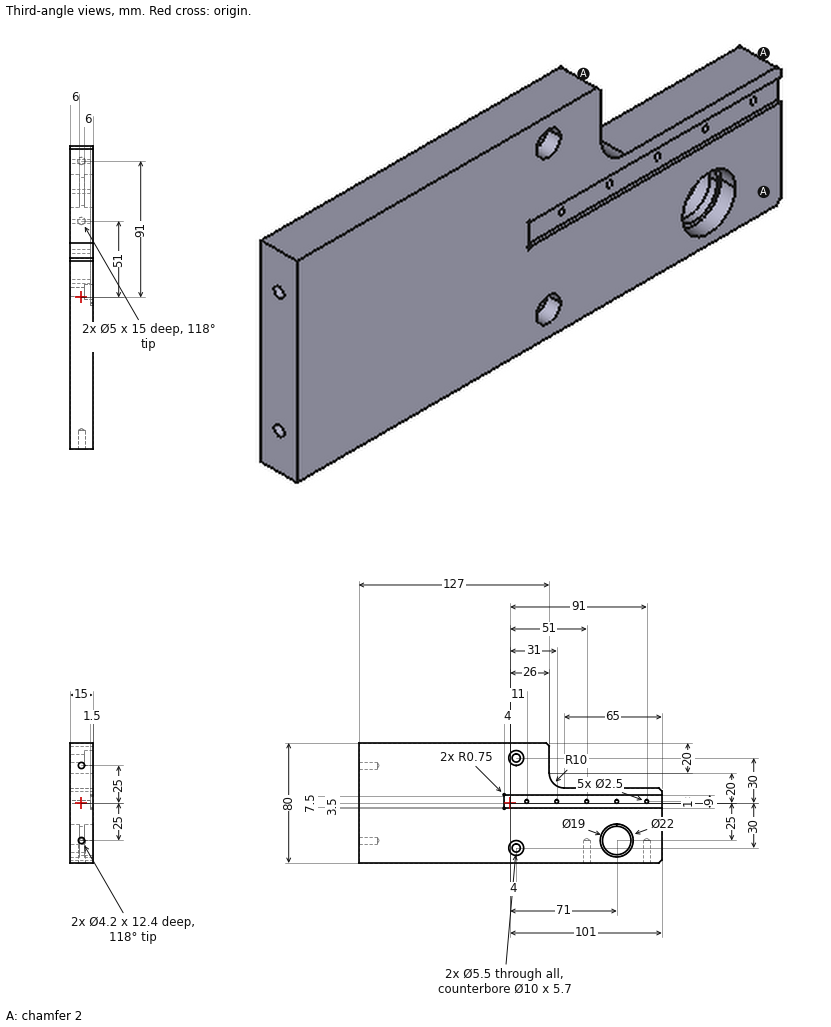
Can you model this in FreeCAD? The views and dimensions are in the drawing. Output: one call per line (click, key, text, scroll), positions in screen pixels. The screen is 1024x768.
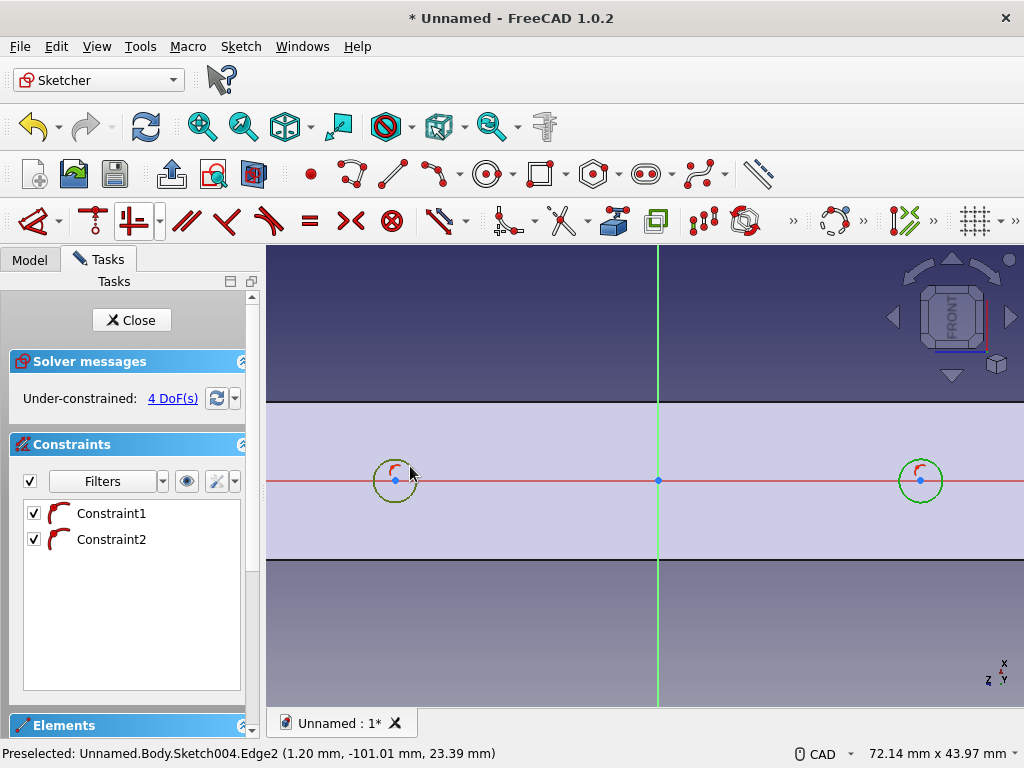
key(e)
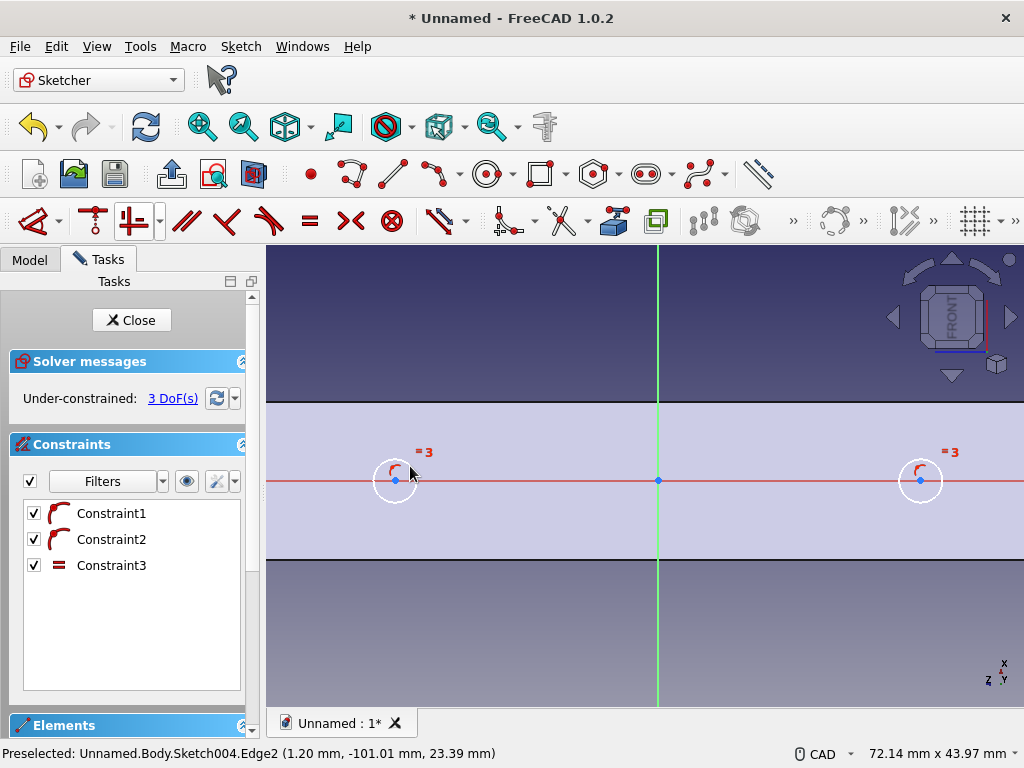
click(32, 222)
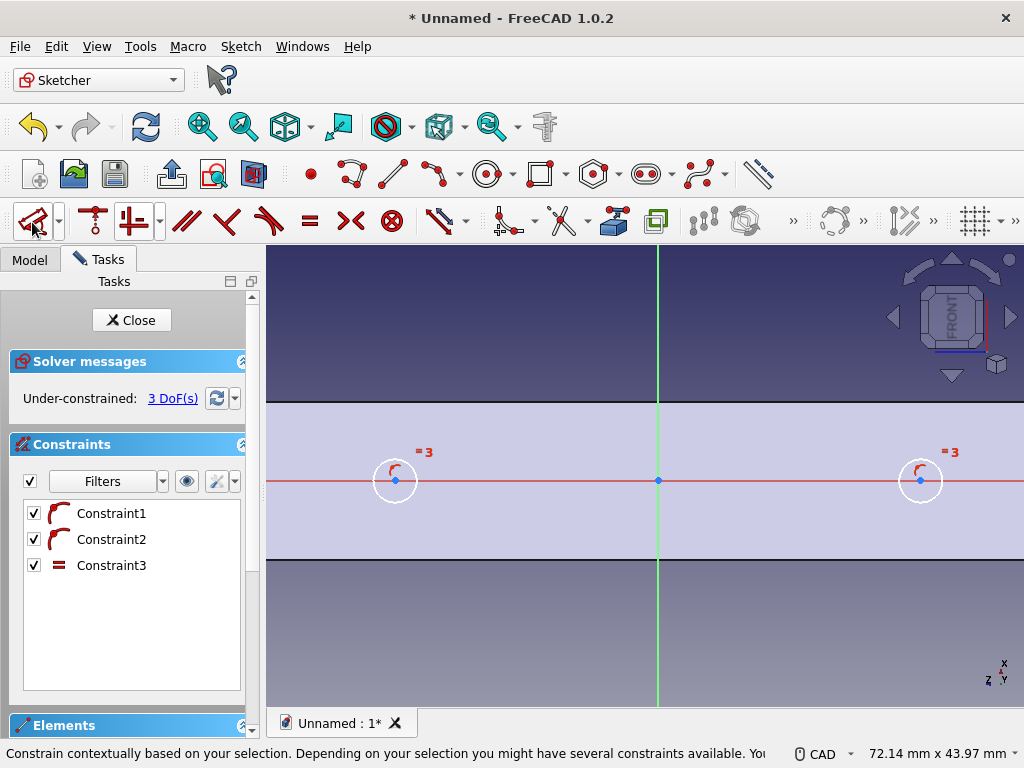
scroll(410, 466, down, 2)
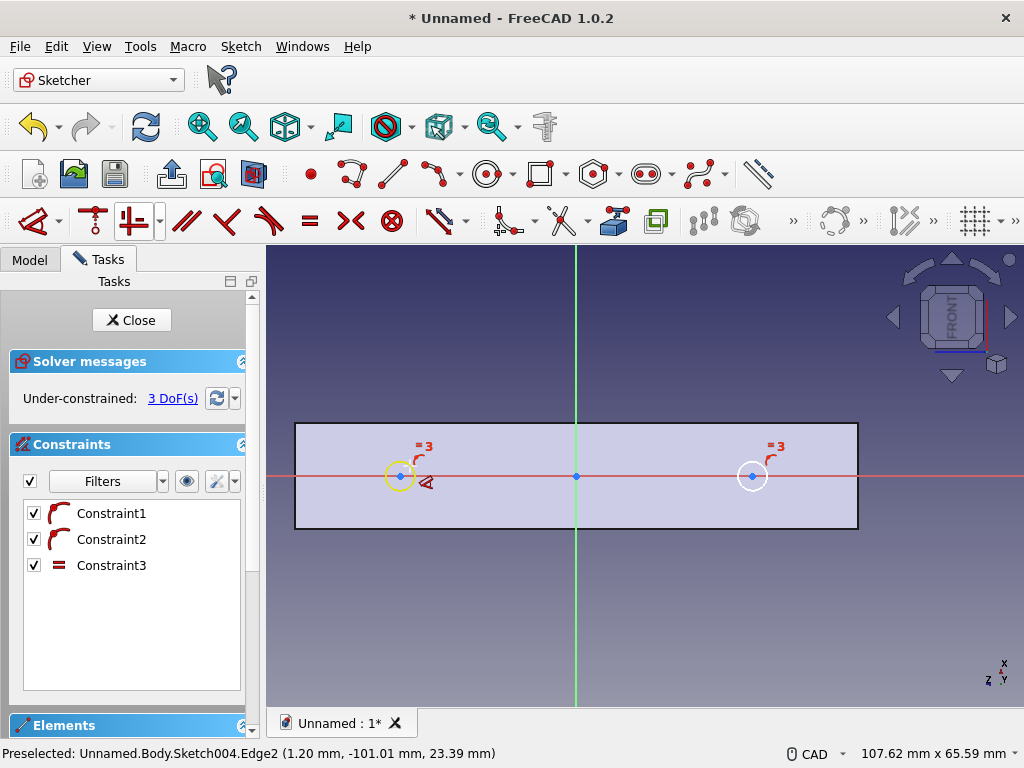
scroll(763, 466, up, 2)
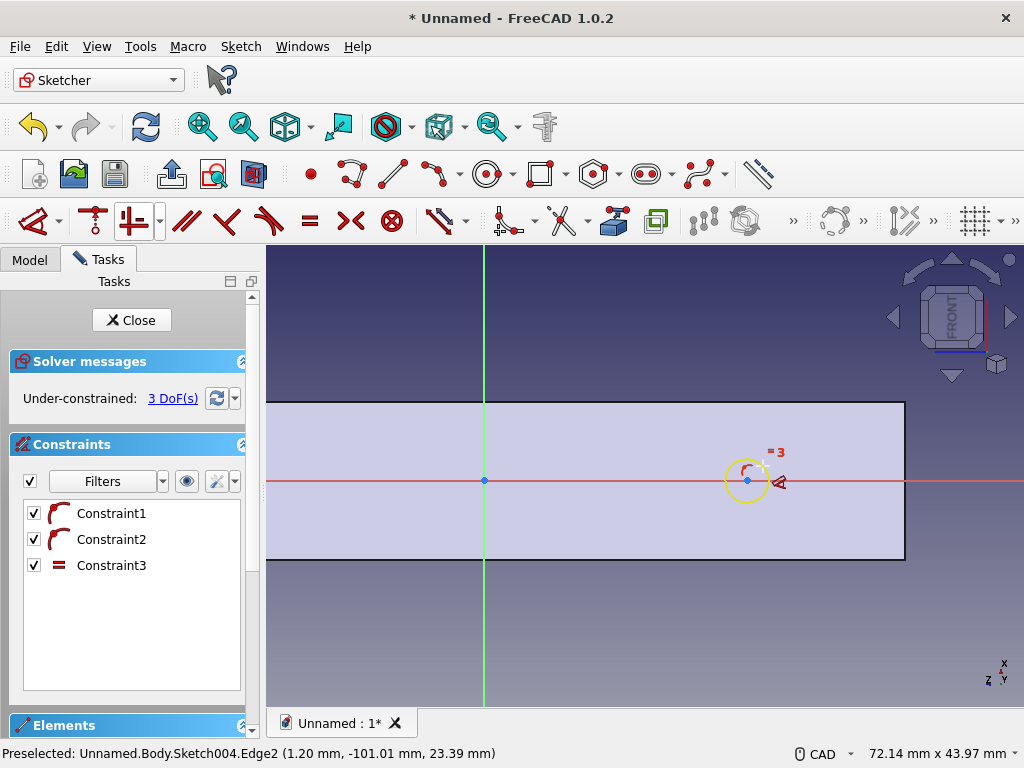
click(762, 466)
click(785, 443)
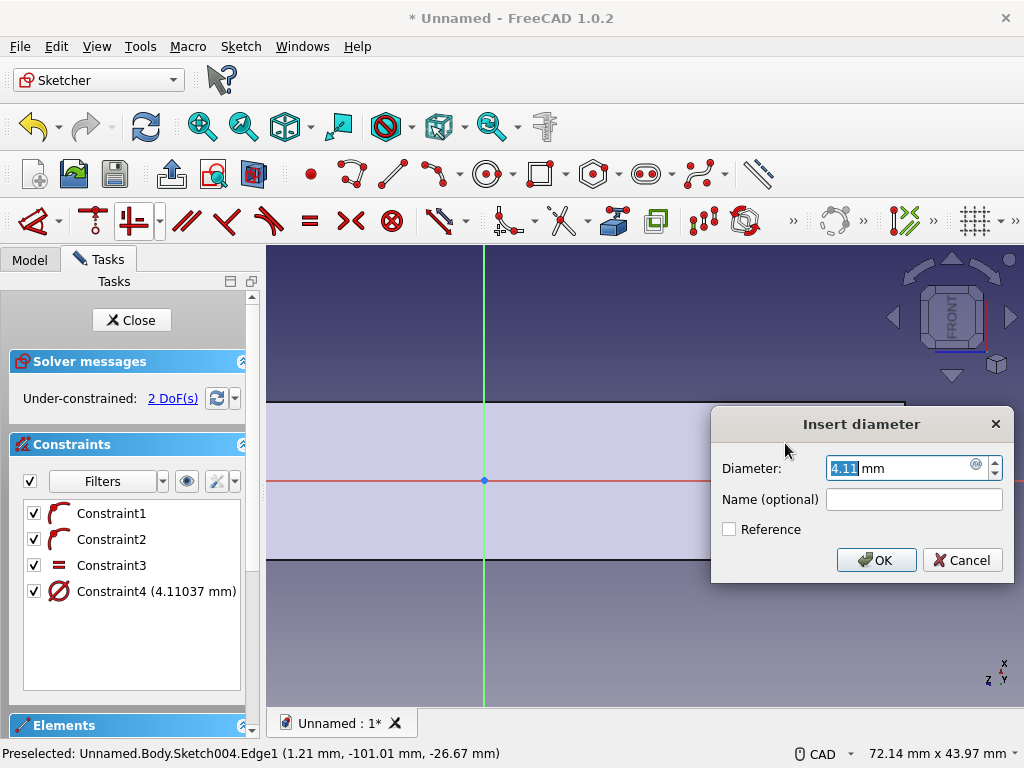
text(4.2)
key(Return)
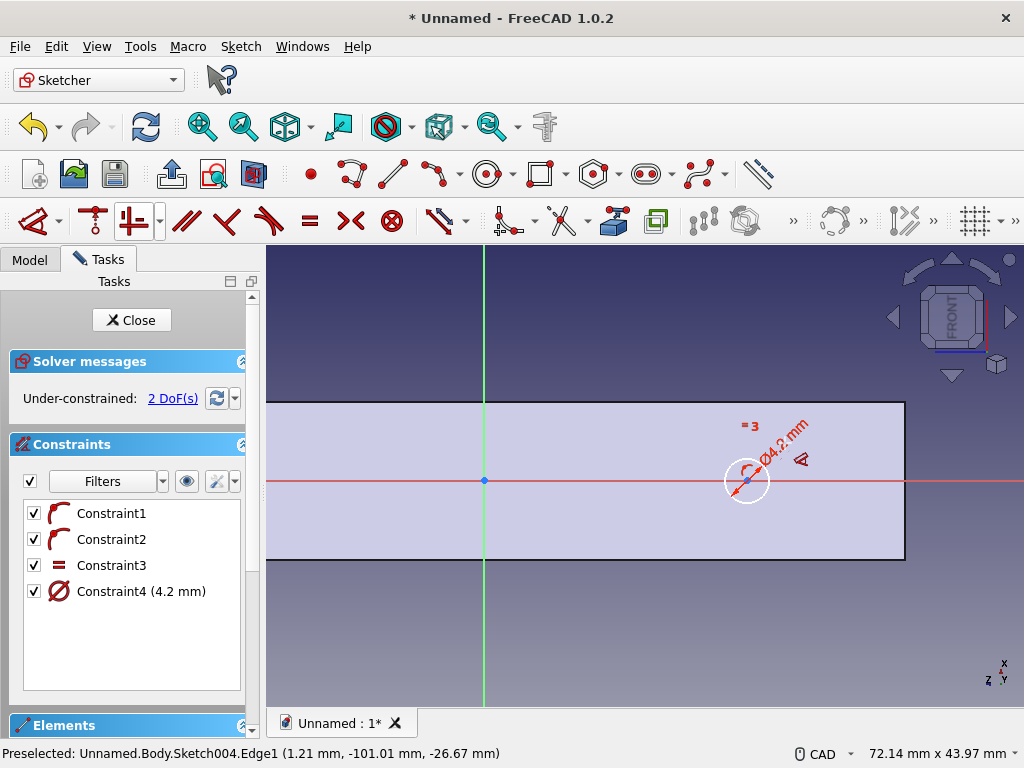
click(747, 481)
click(616, 515)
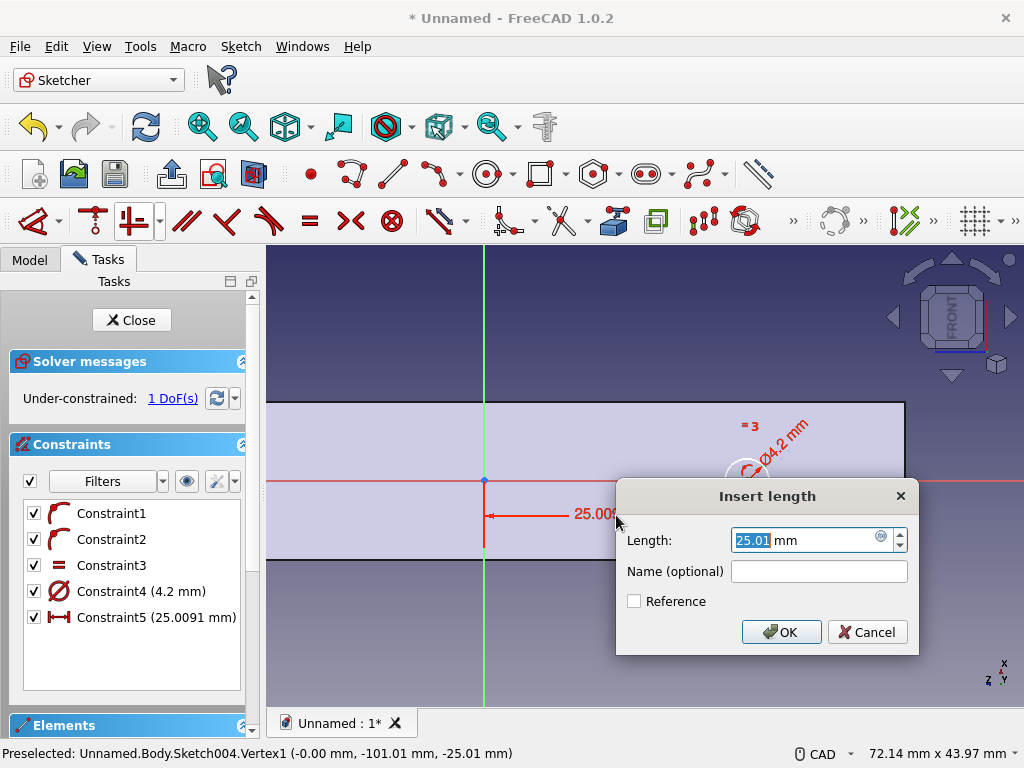
text(25)
key(Return)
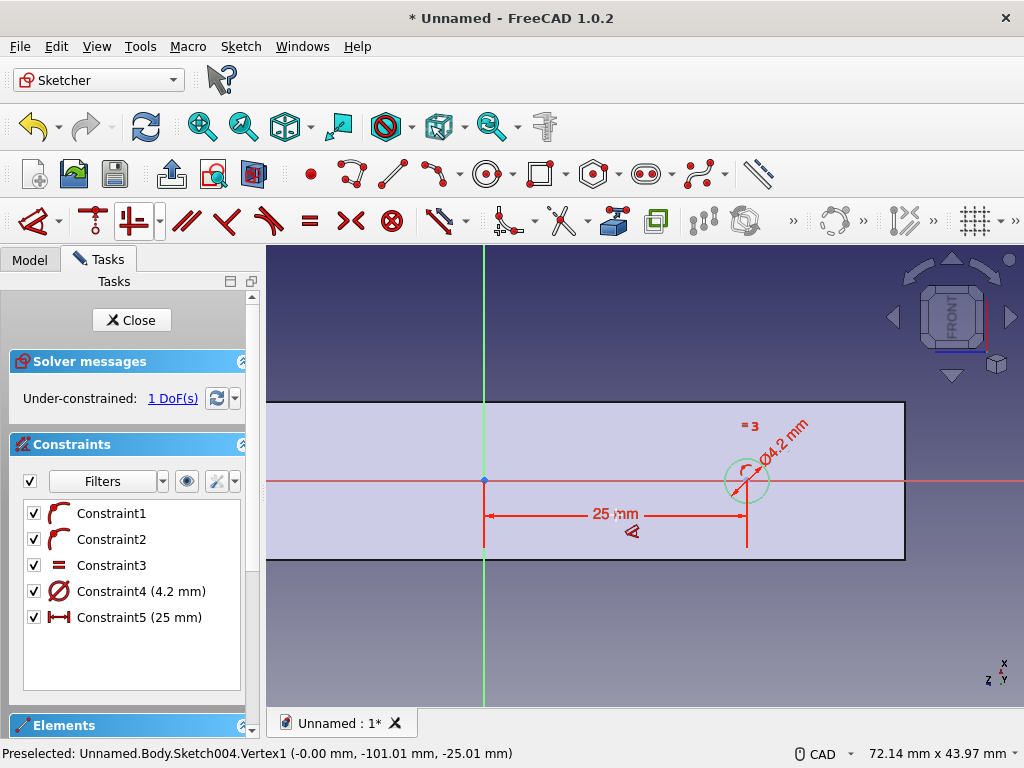
scroll(764, 466, down, 2)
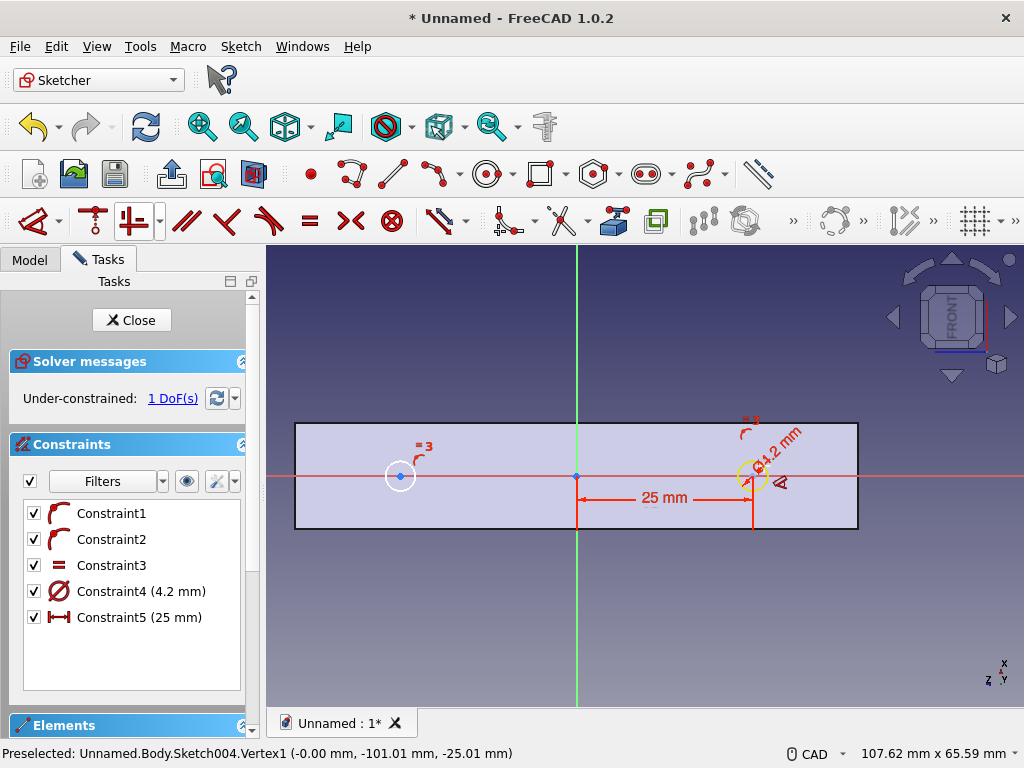
click(400, 476)
click(489, 510)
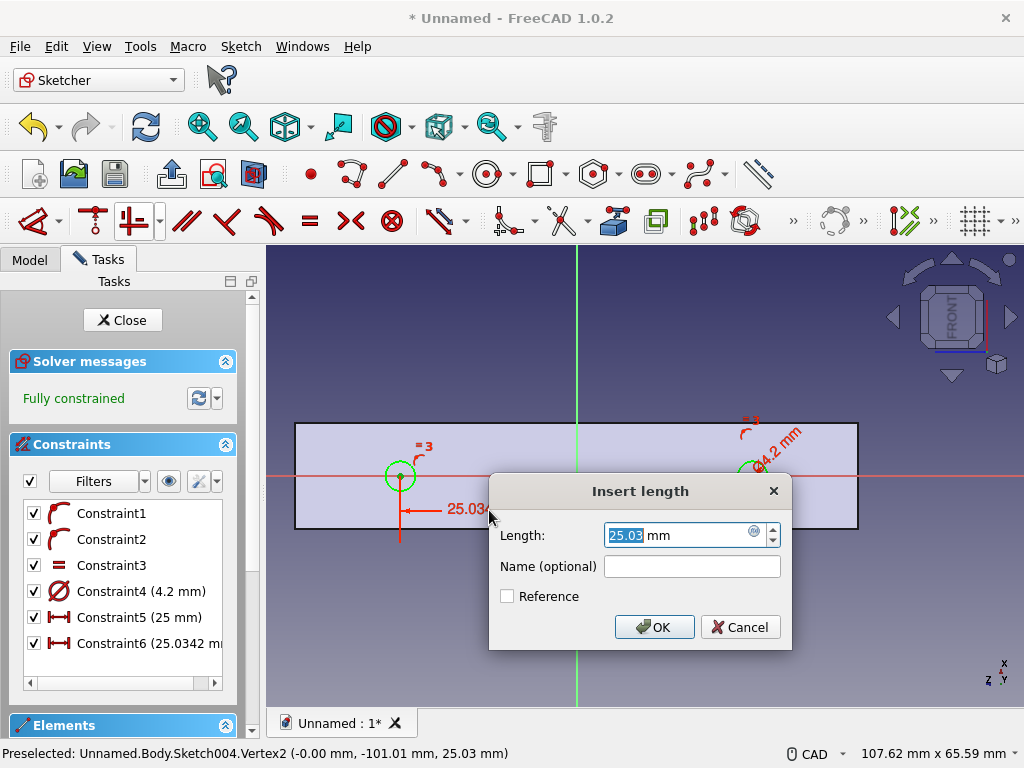
text(25)
key(Return)
key(Escape)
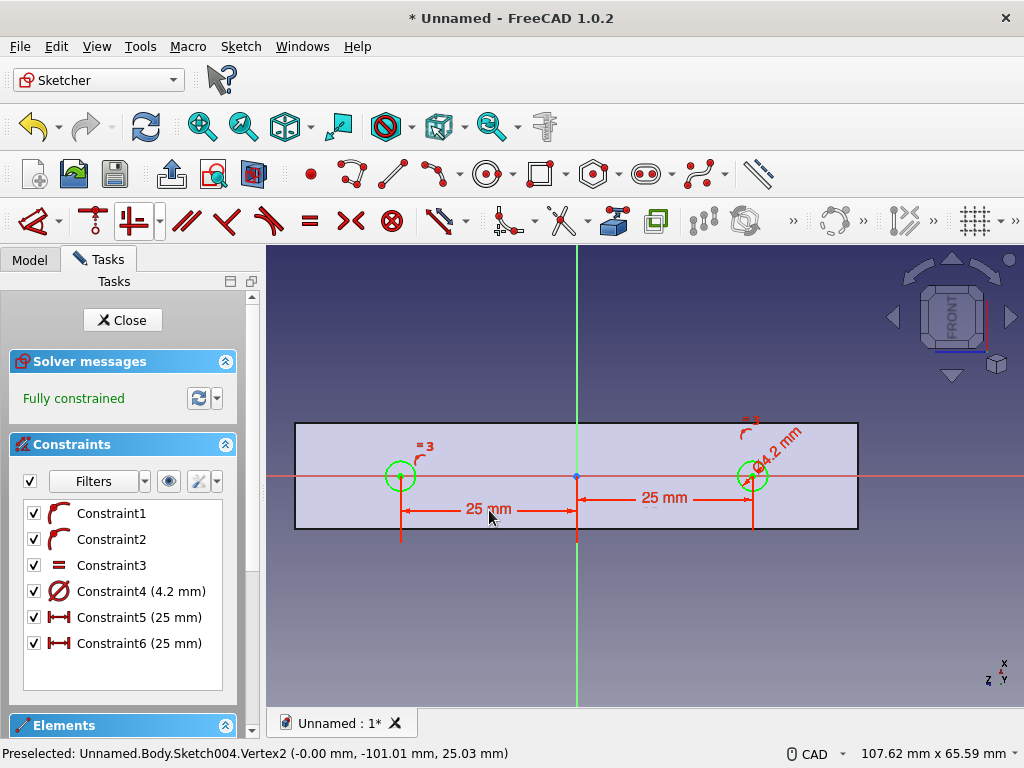
click(123, 320)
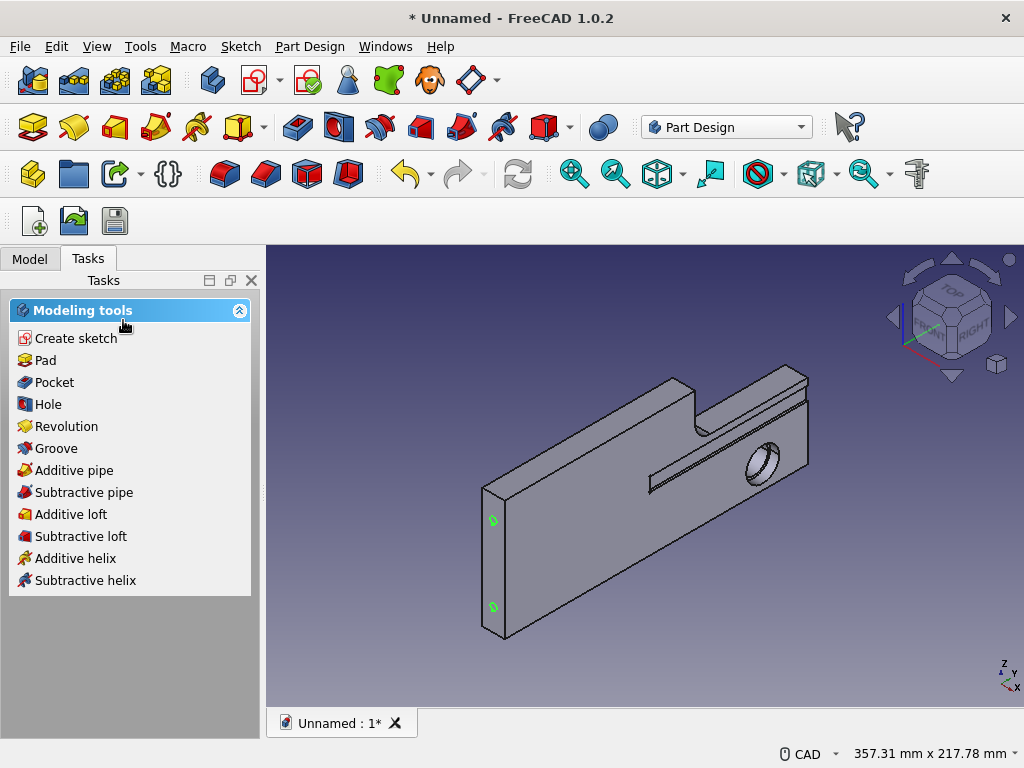
click(339, 128)